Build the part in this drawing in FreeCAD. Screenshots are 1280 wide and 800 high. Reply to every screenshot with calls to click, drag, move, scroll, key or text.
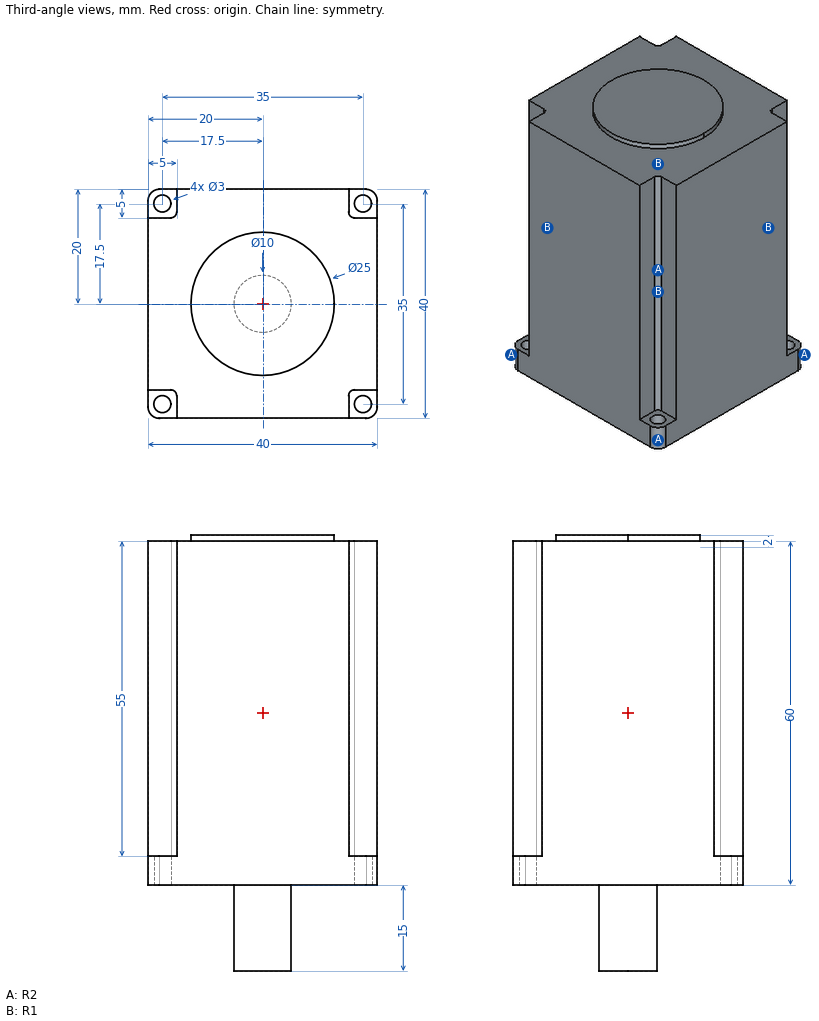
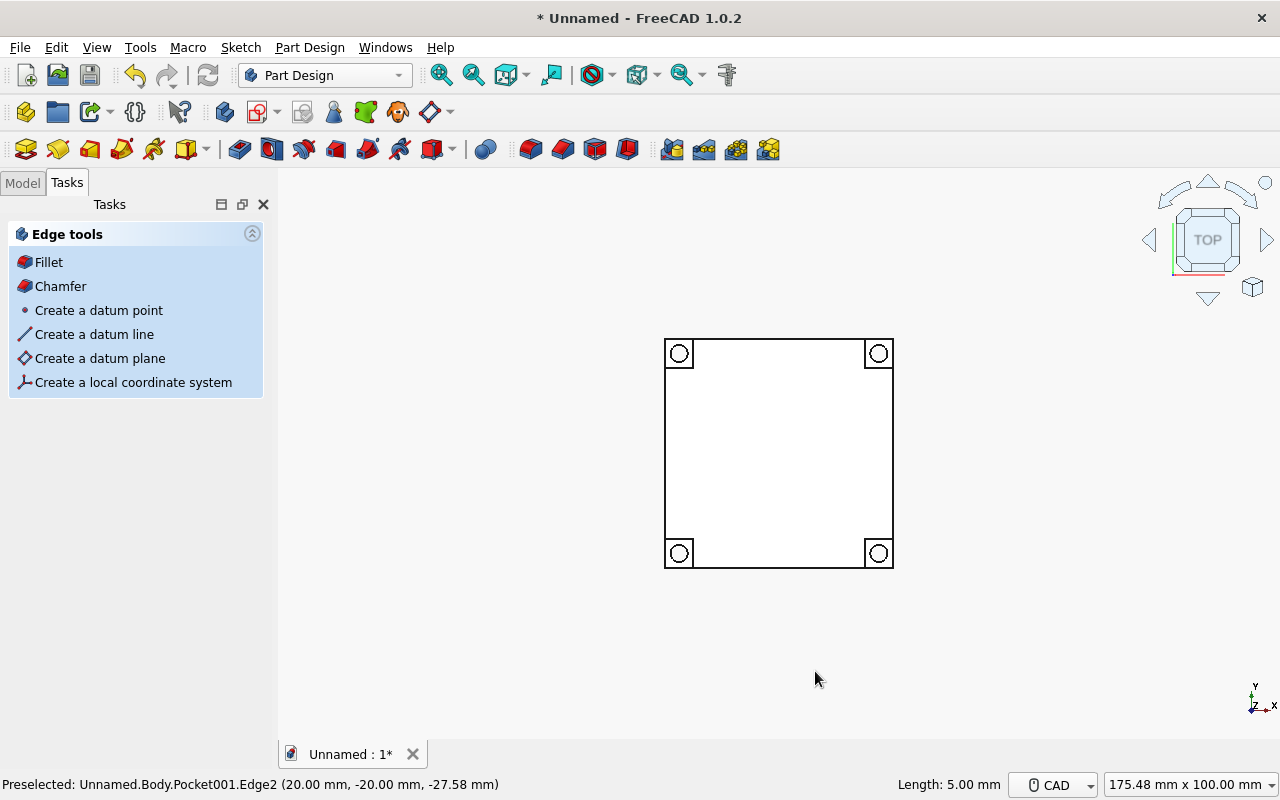
click(442, 76)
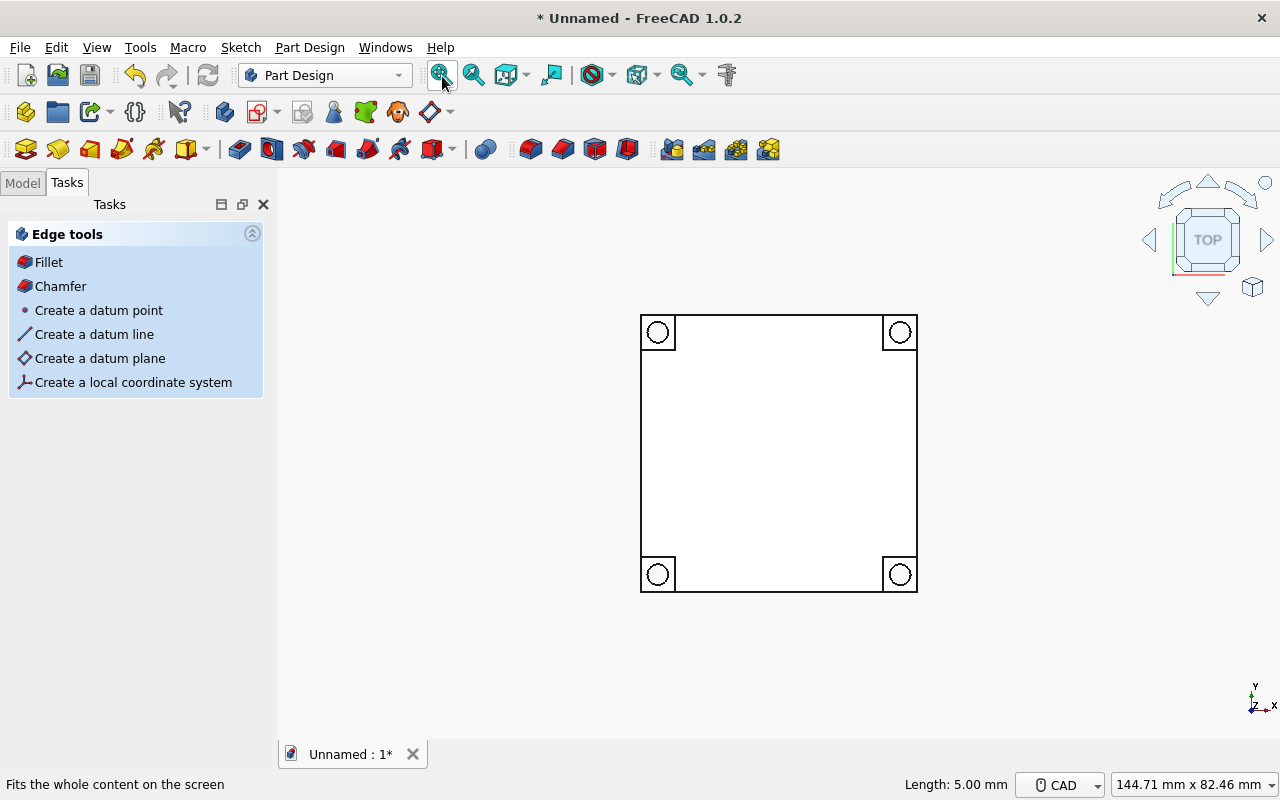
key(1)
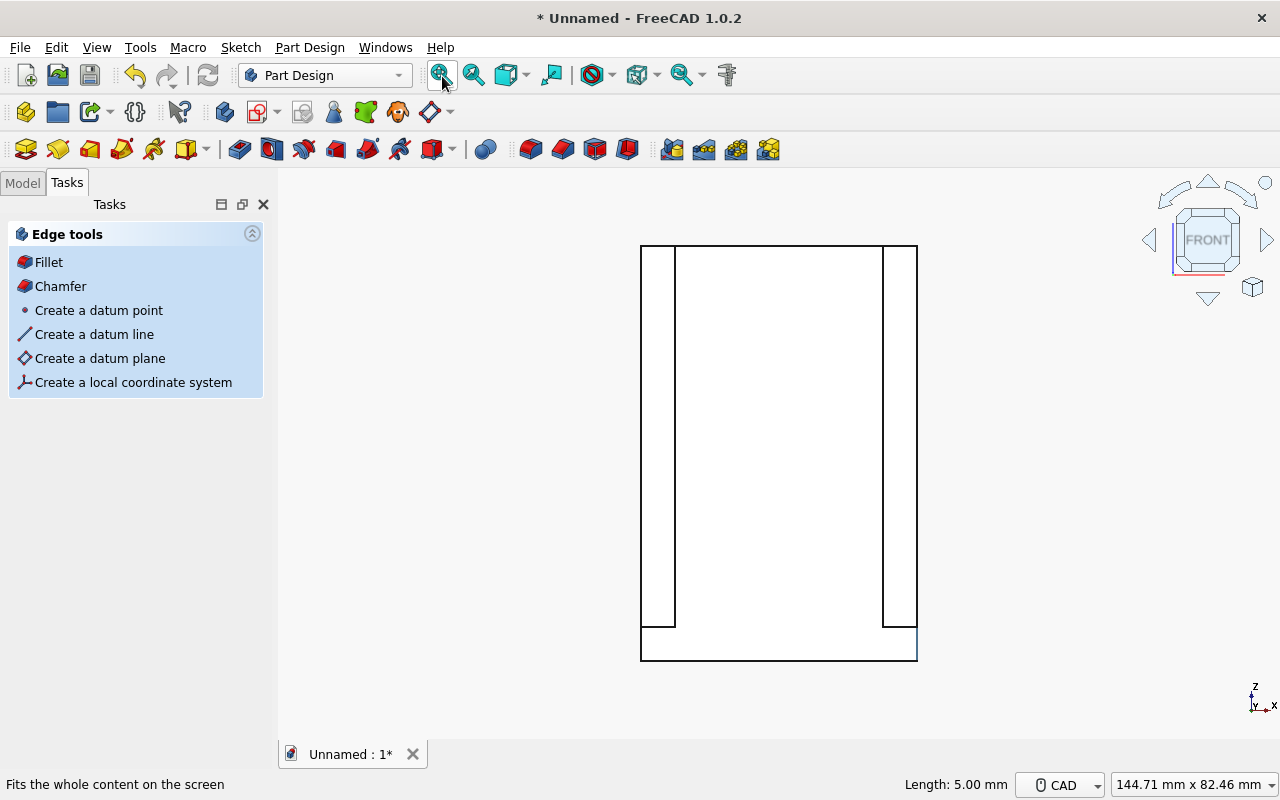
click(641, 643, ctrl)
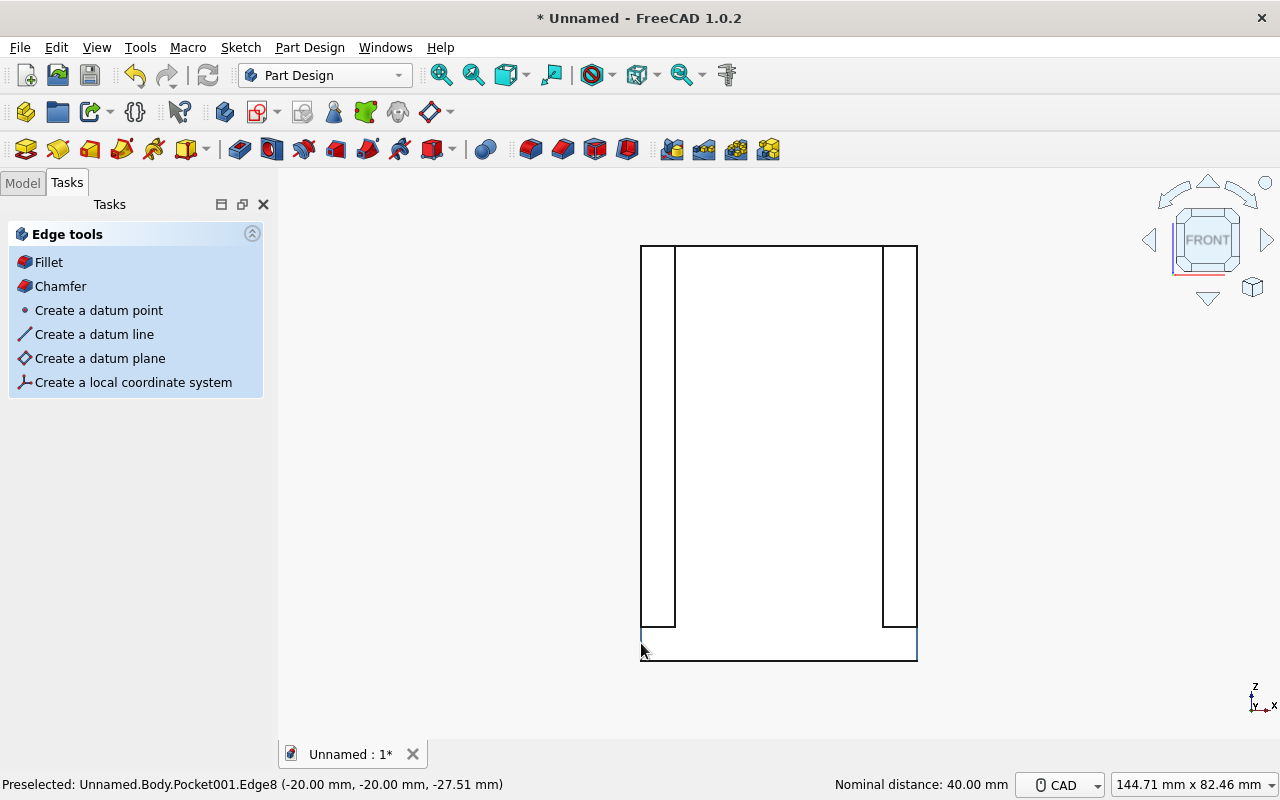
key(3)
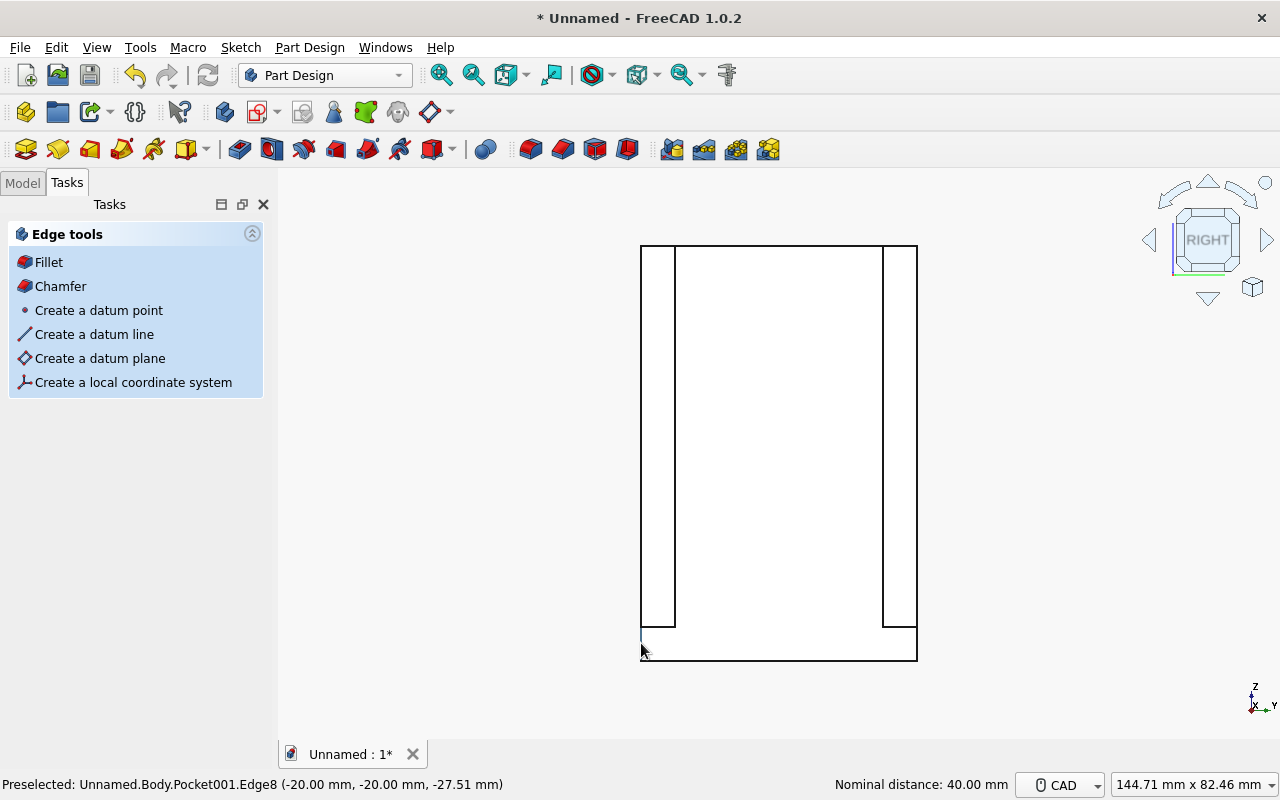
click(917, 643, ctrl)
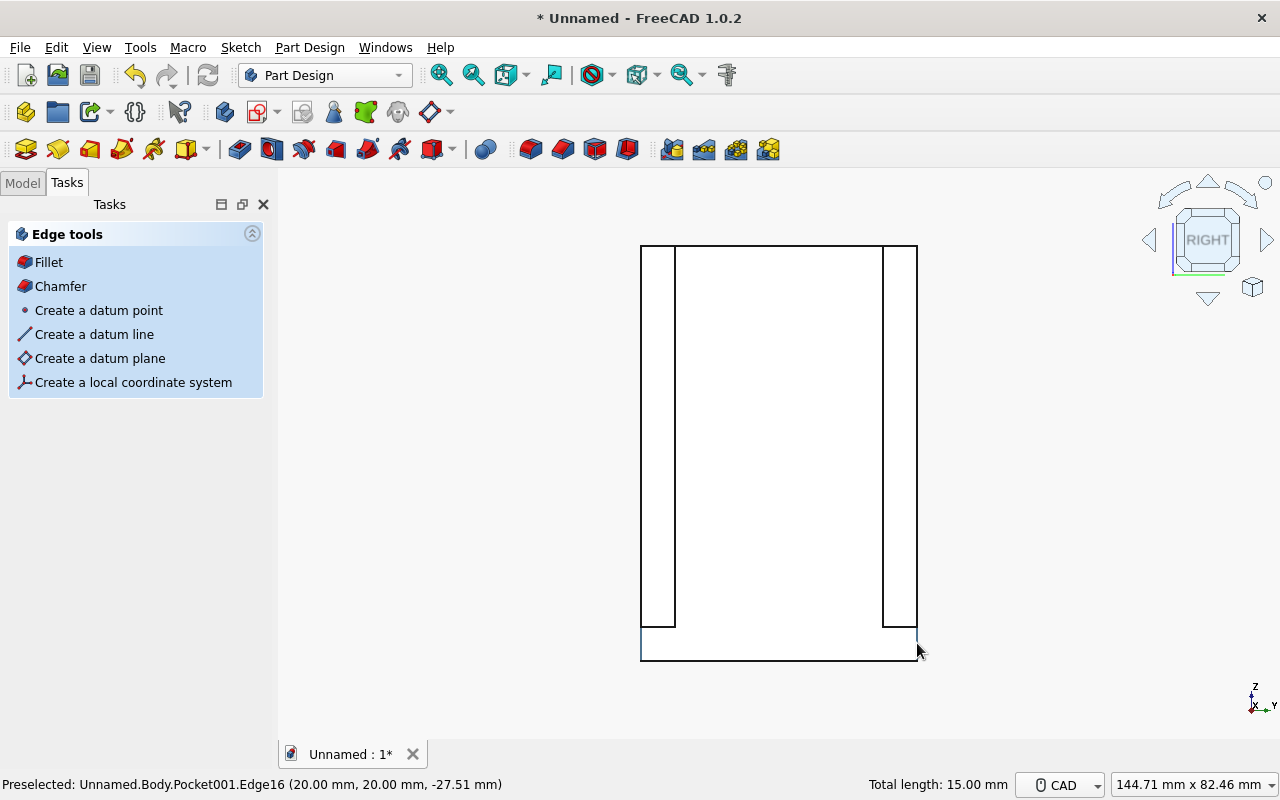
key(5)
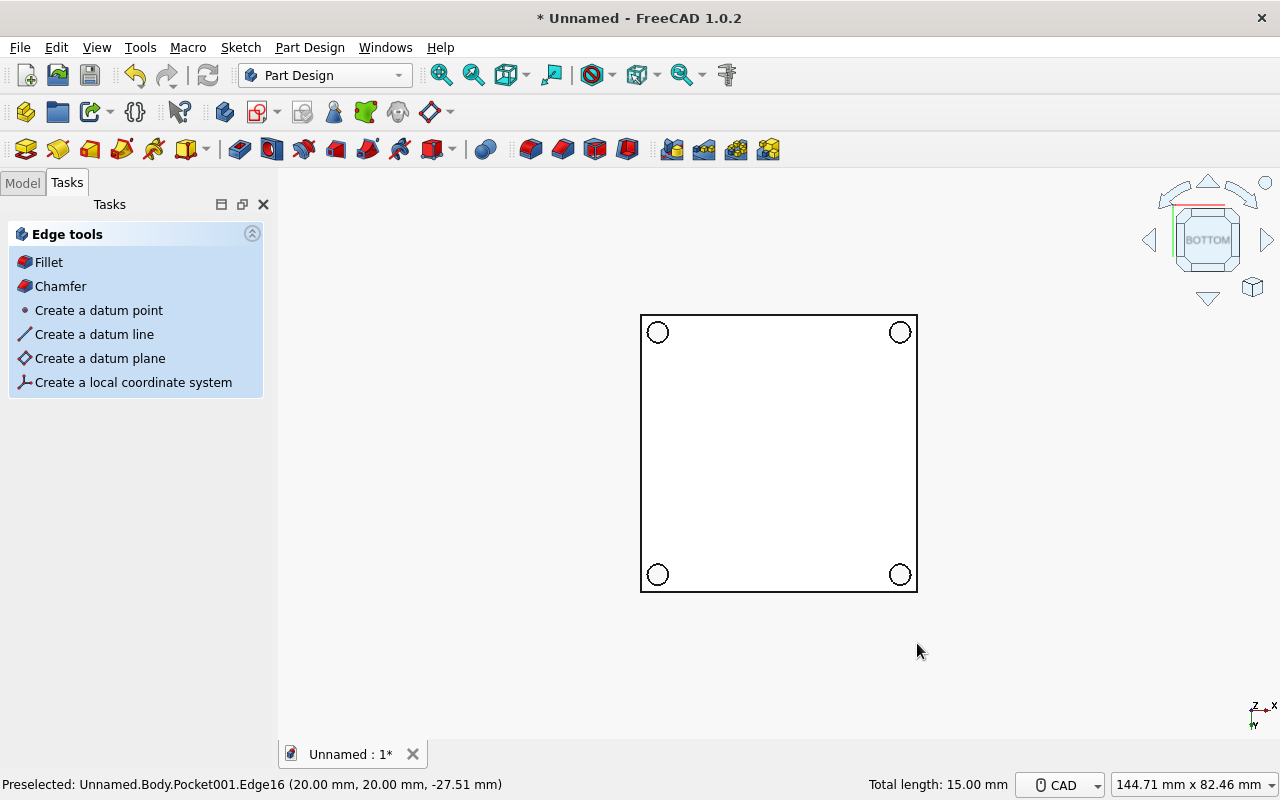
key(4)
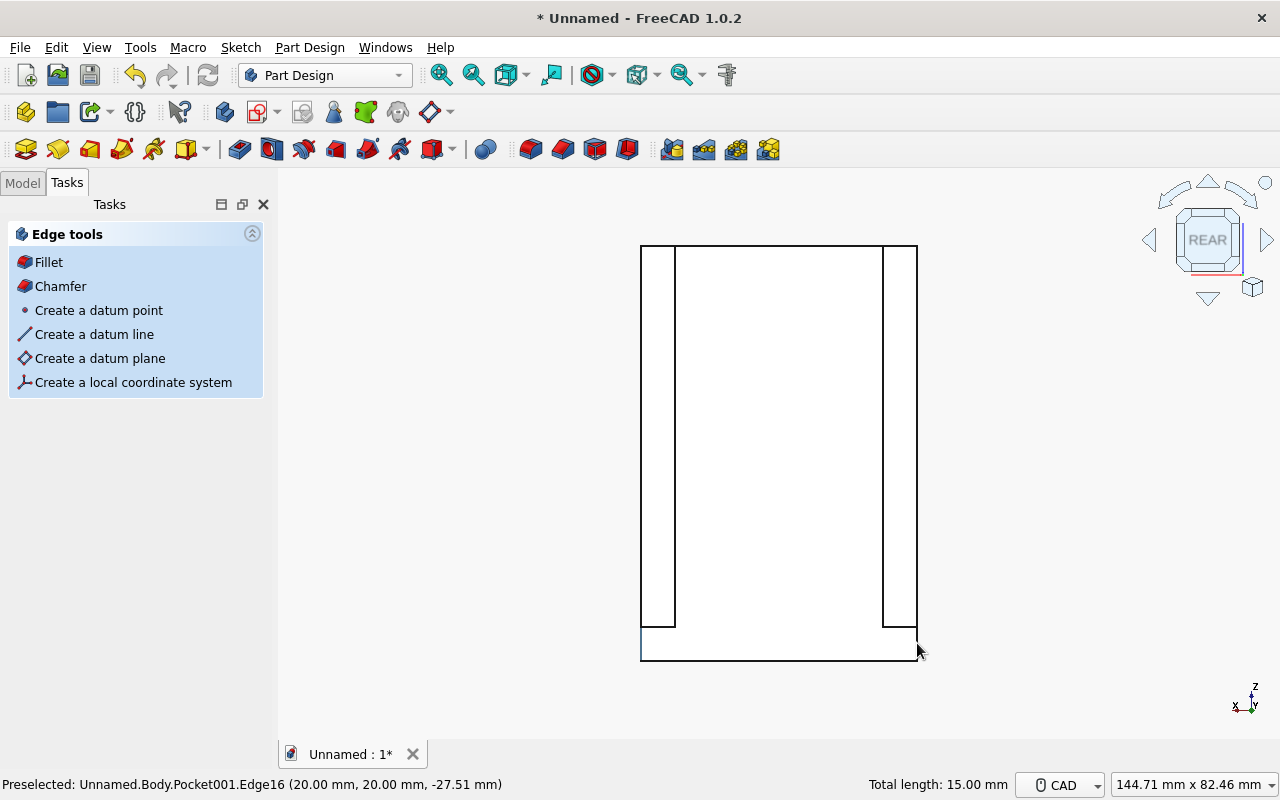
click(917, 643, ctrl)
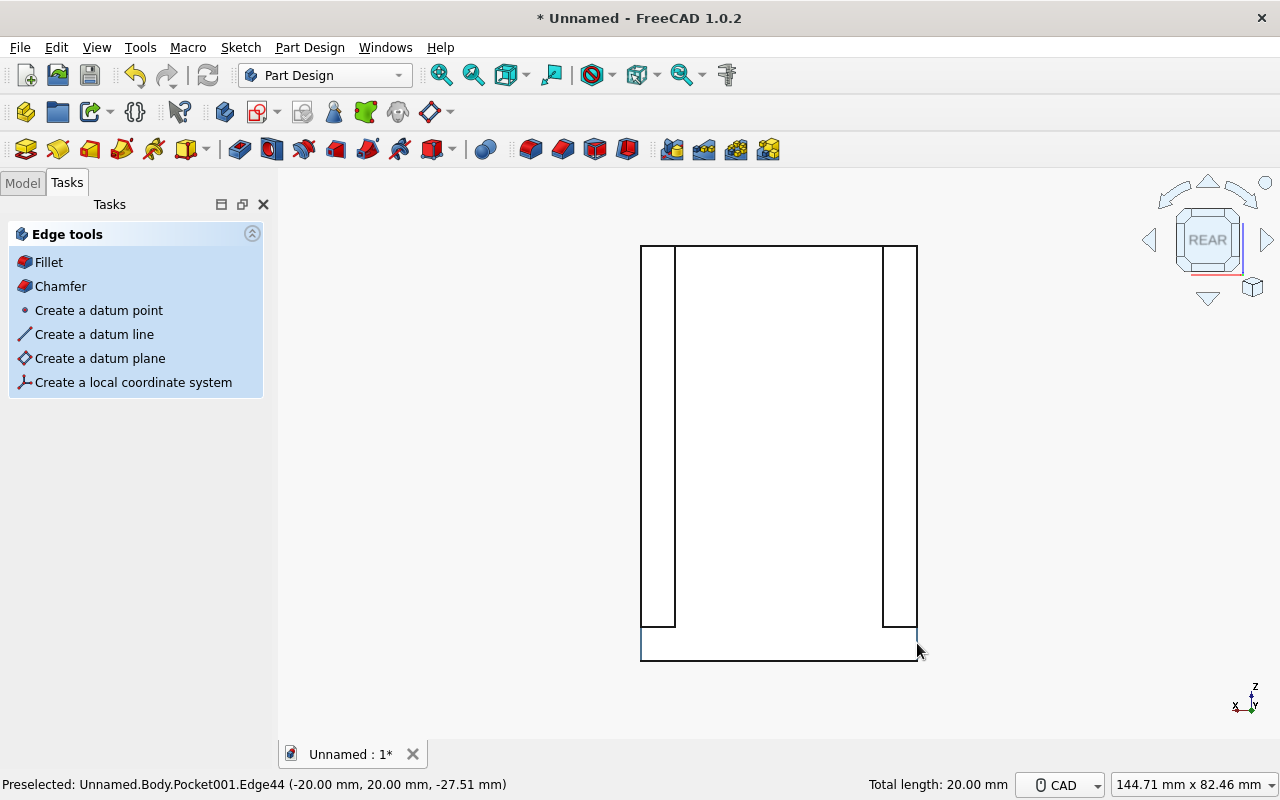
click(532, 150)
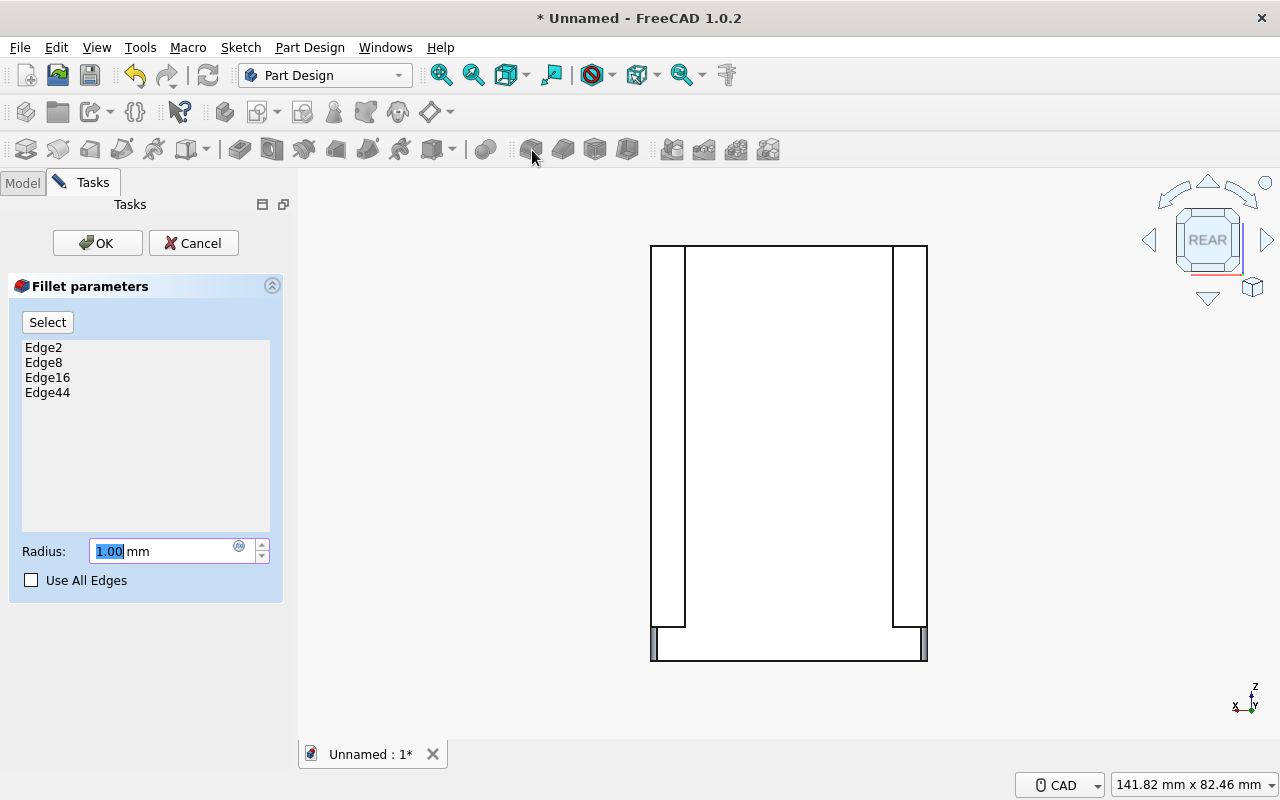
text(2)
key(Tab)